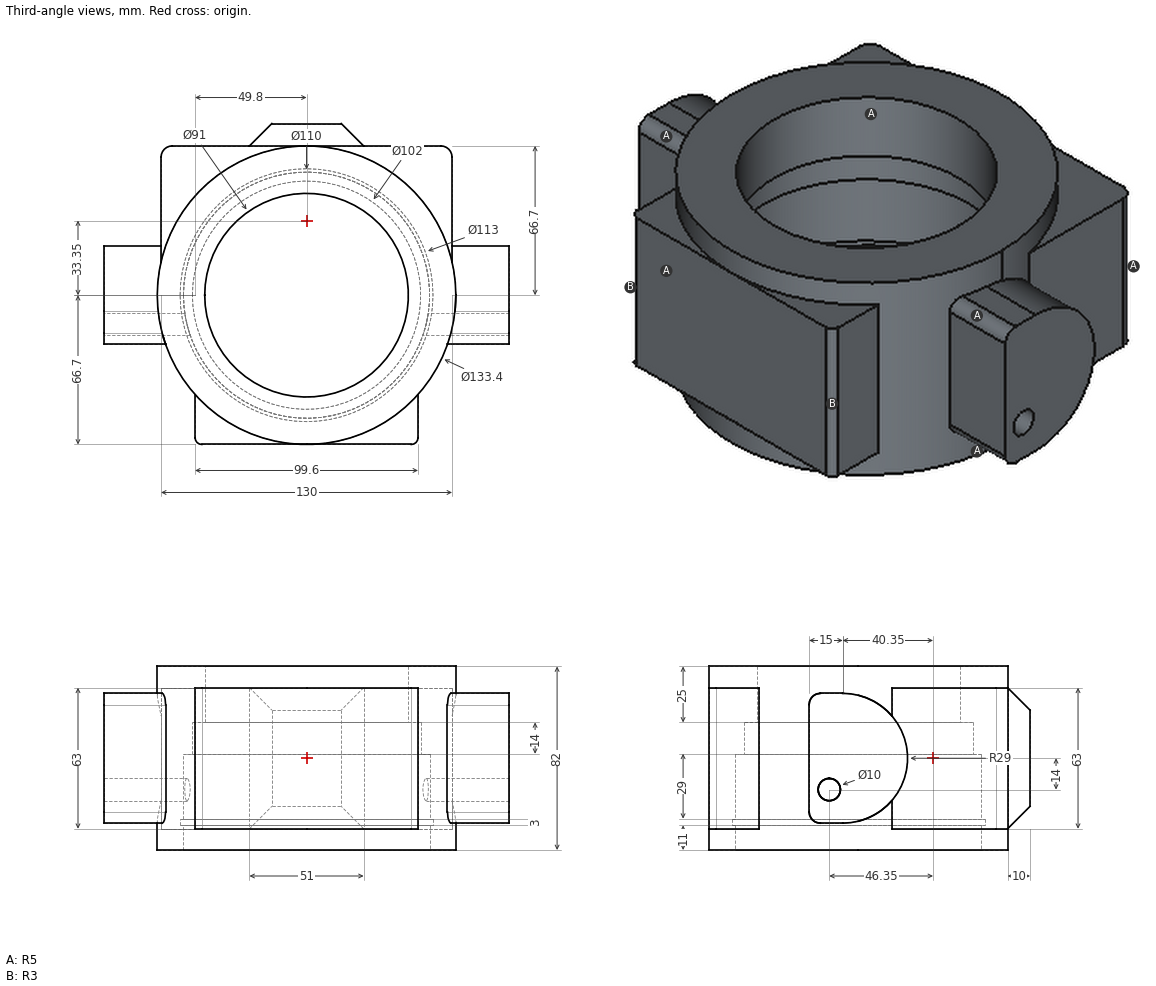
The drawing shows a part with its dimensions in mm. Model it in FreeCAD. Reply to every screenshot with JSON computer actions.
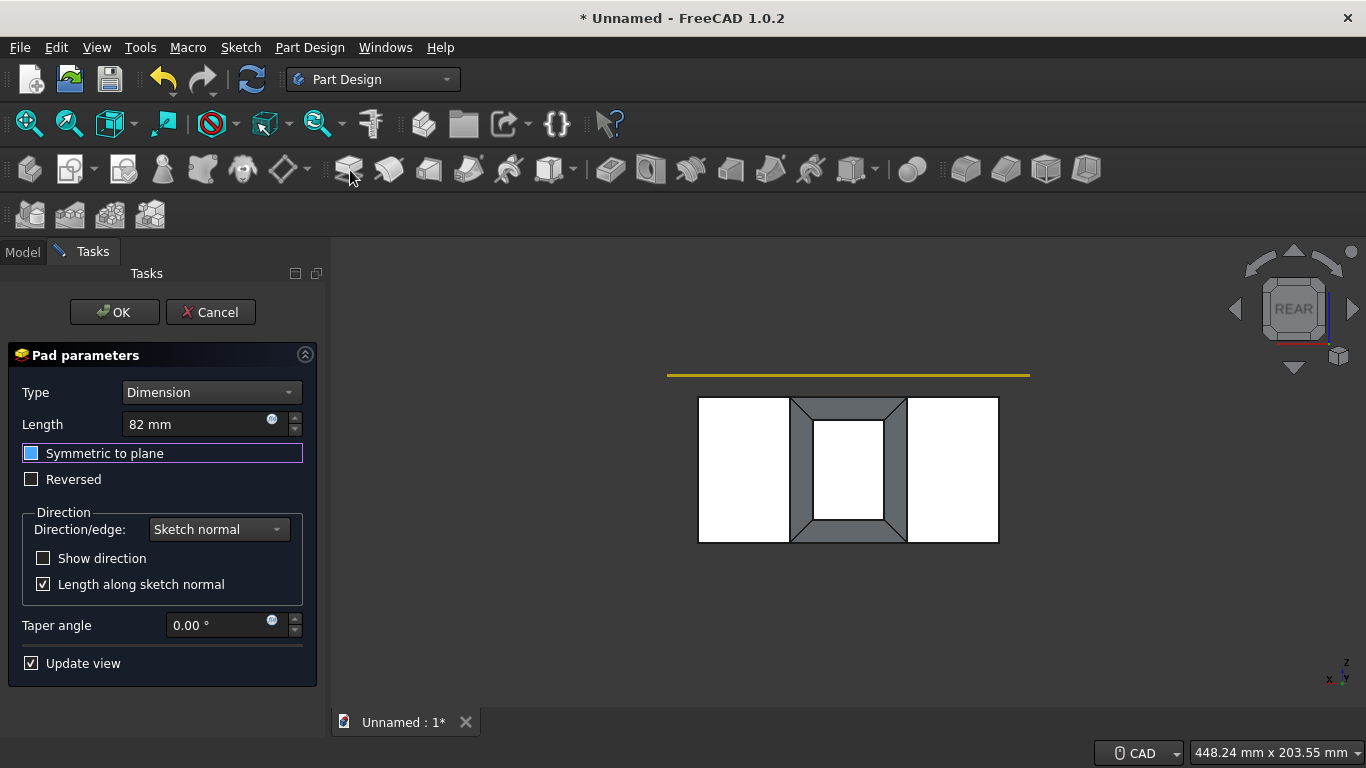
{"action": "left_click", "coordinate": [30, 479]}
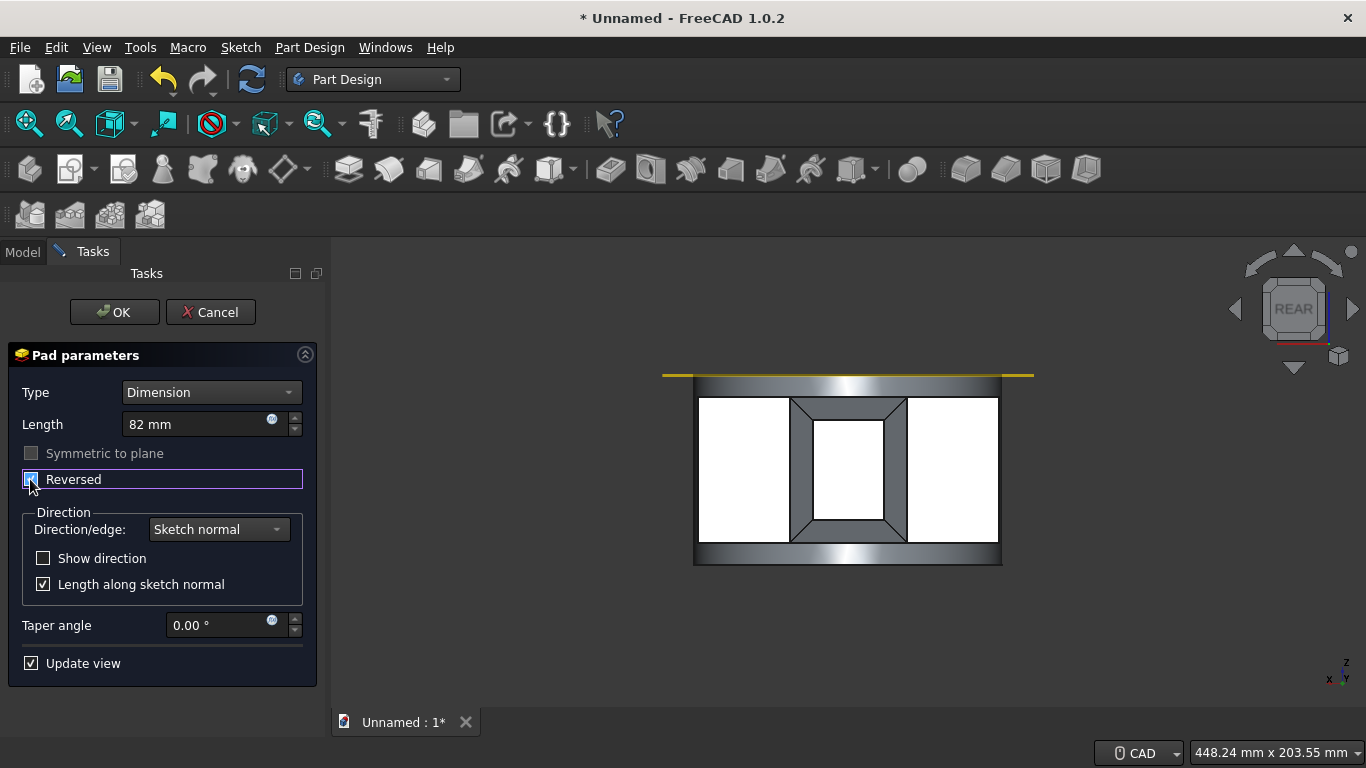
{"action": "left_click", "coordinate": [115, 312]}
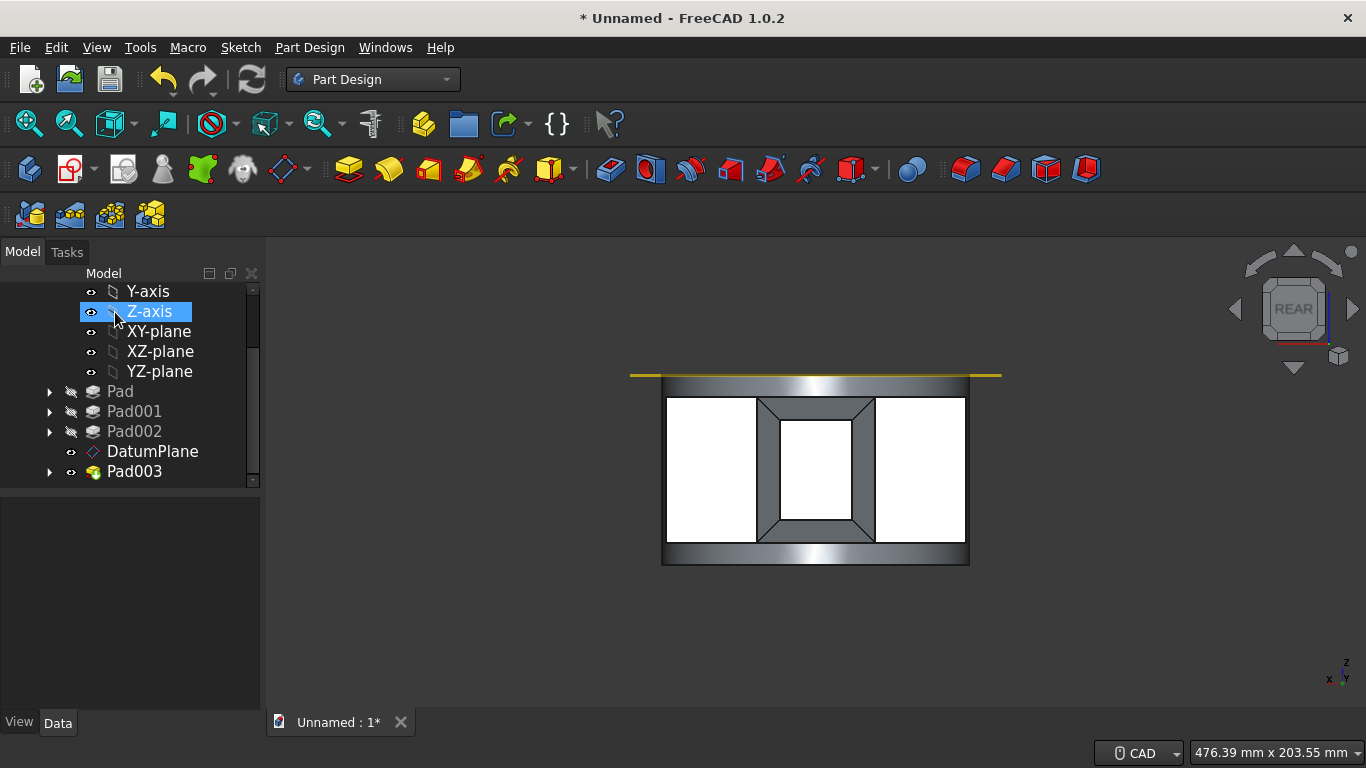
{"action": "left_click", "coordinate": [116, 452]}
{"action": "key", "text": "space"}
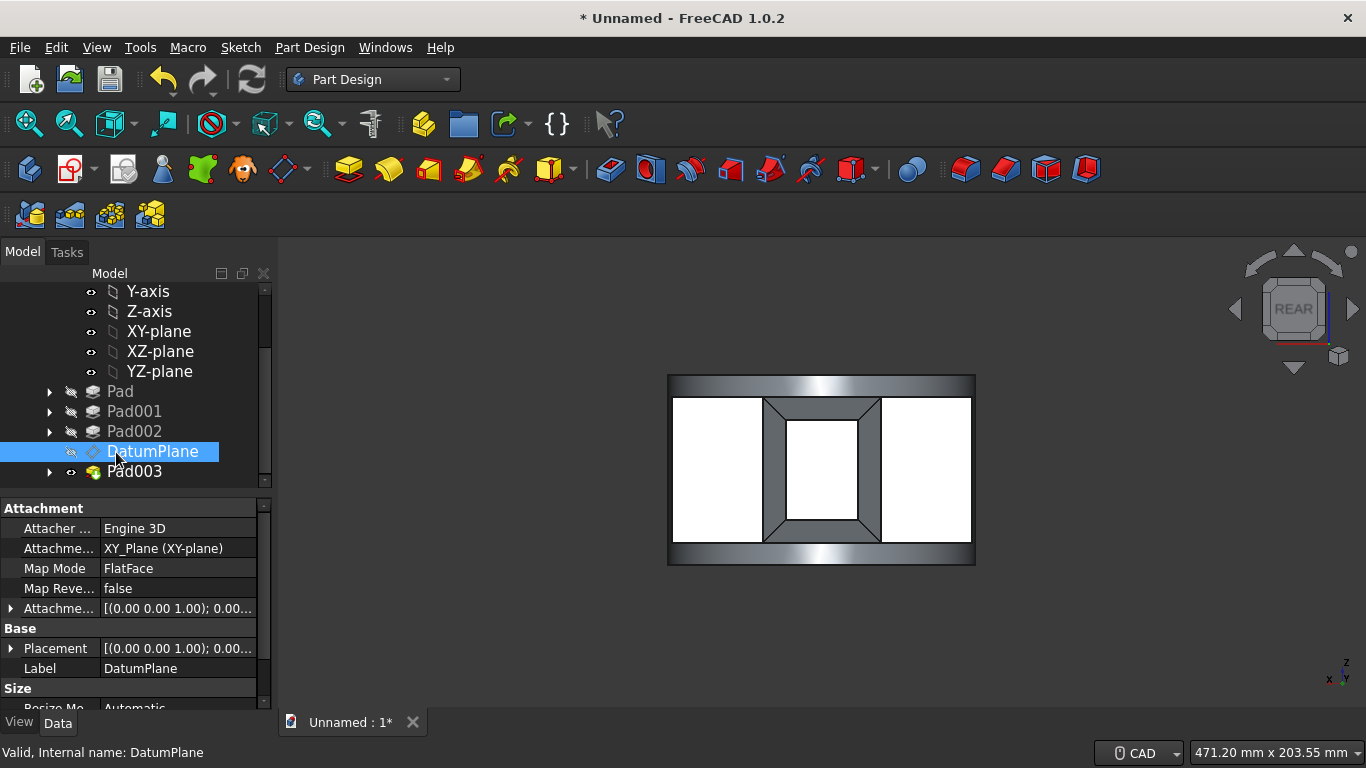
{"action": "key", "text": "v f"}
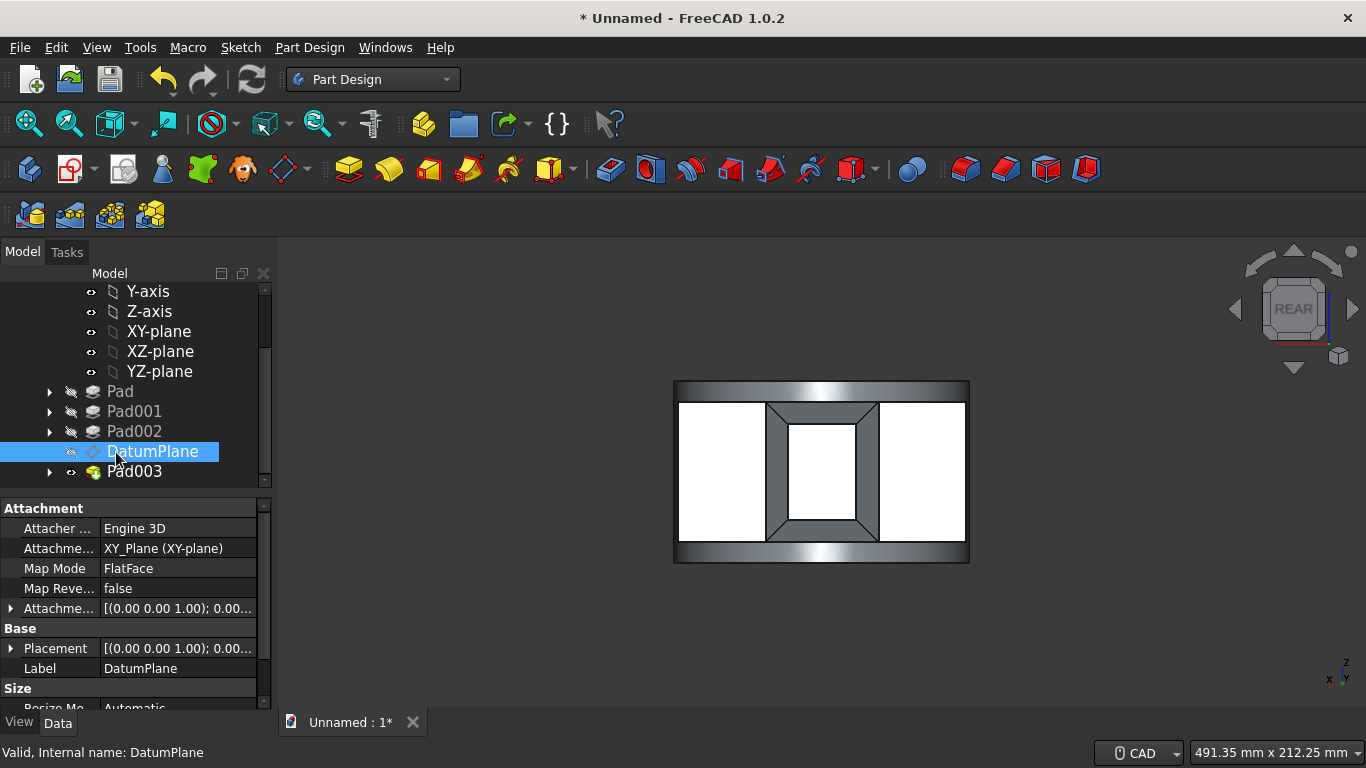
{"action": "key", "text": "5"}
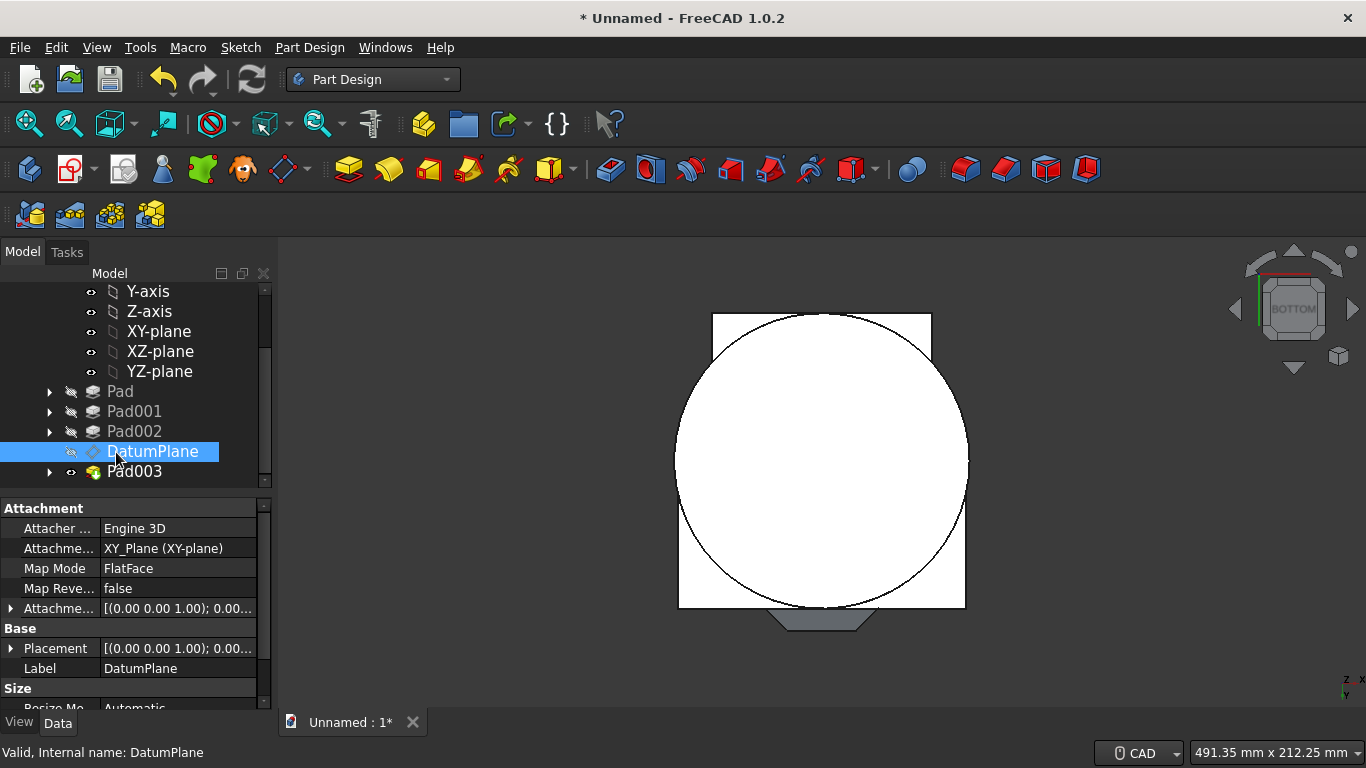
{"action": "left_click", "coordinate": [822, 460]}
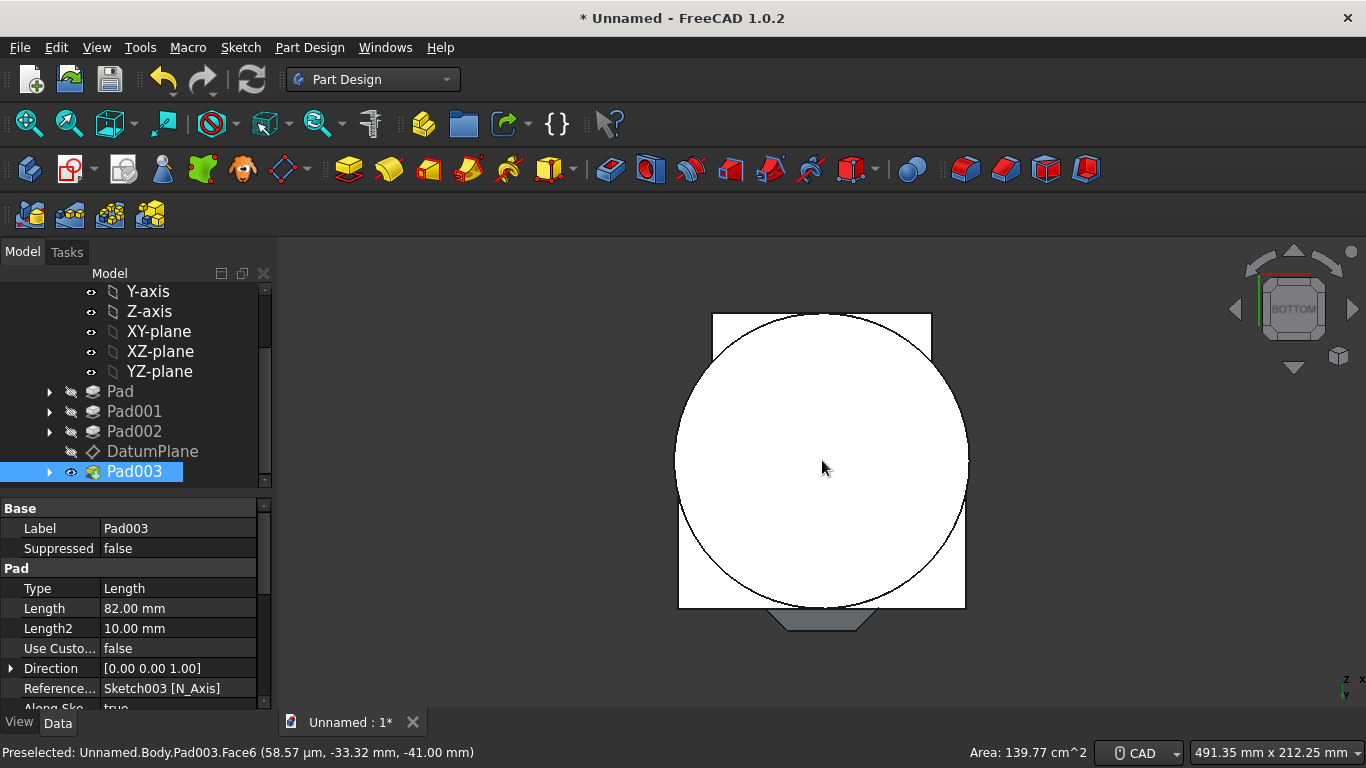
{"action": "left_click", "coordinate": [70, 170]}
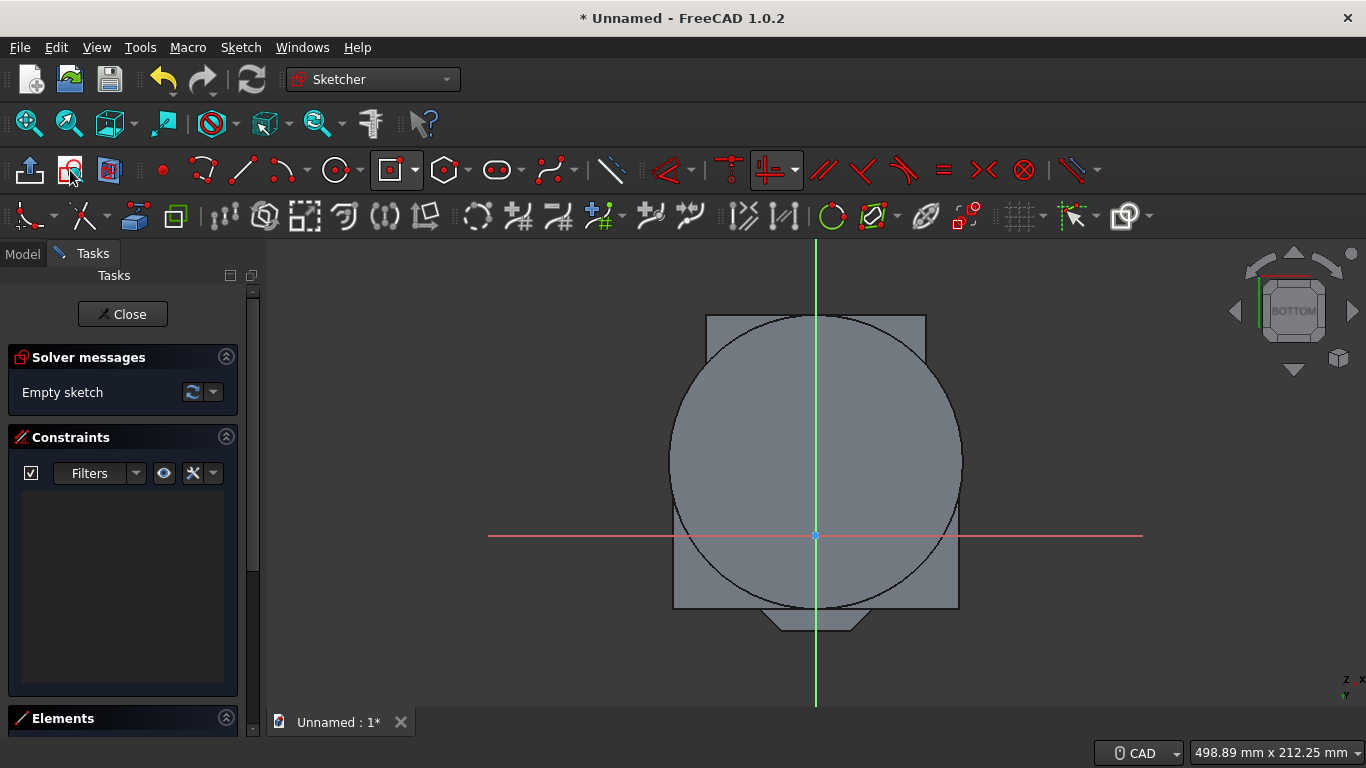
{"action": "left_click", "coordinate": [336, 170]}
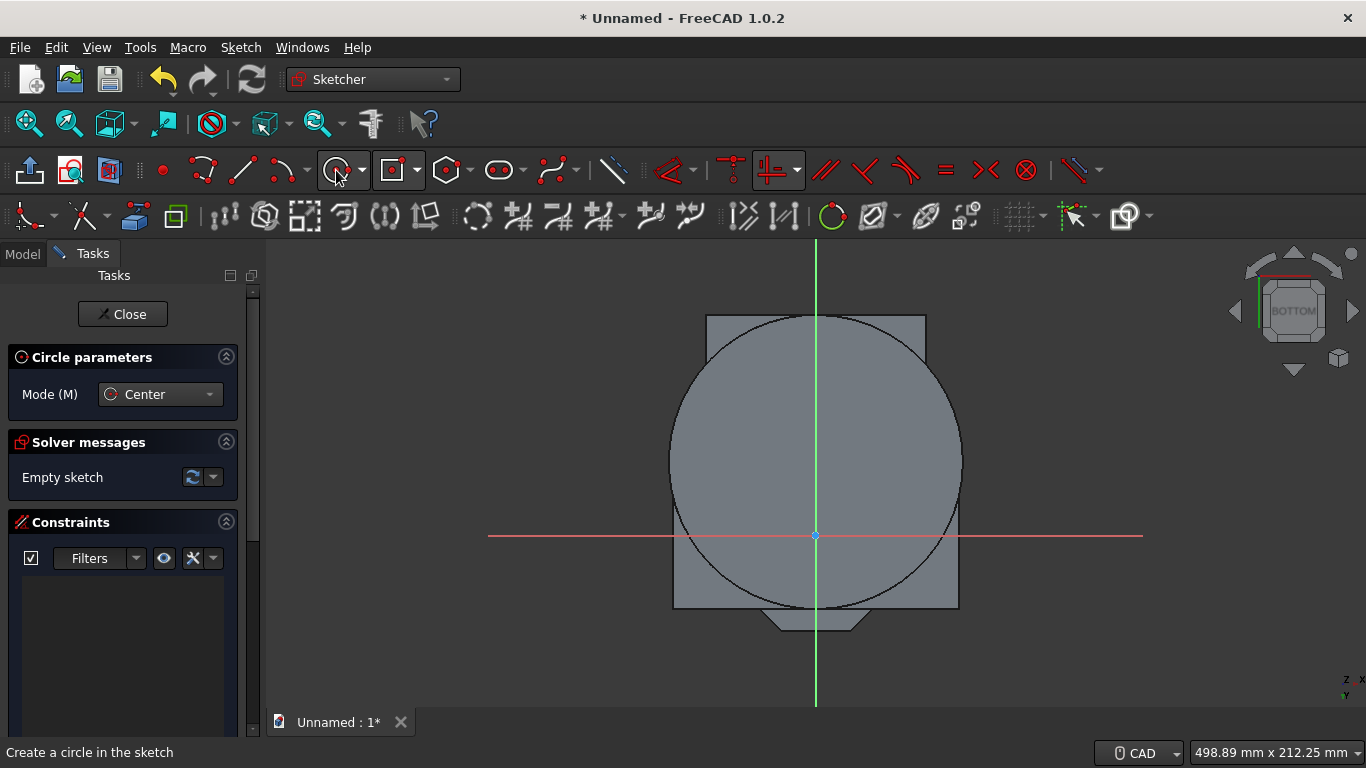
{"action": "left_click", "coordinate": [816, 462]}
{"action": "left_click", "coordinate": [902, 376]}
{"action": "key", "text": "Escape"}